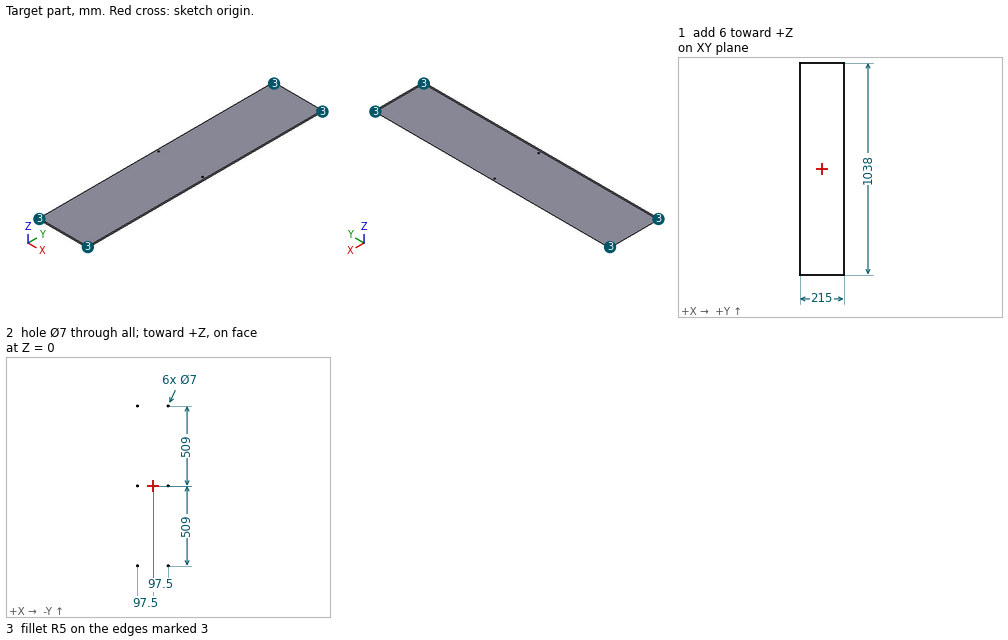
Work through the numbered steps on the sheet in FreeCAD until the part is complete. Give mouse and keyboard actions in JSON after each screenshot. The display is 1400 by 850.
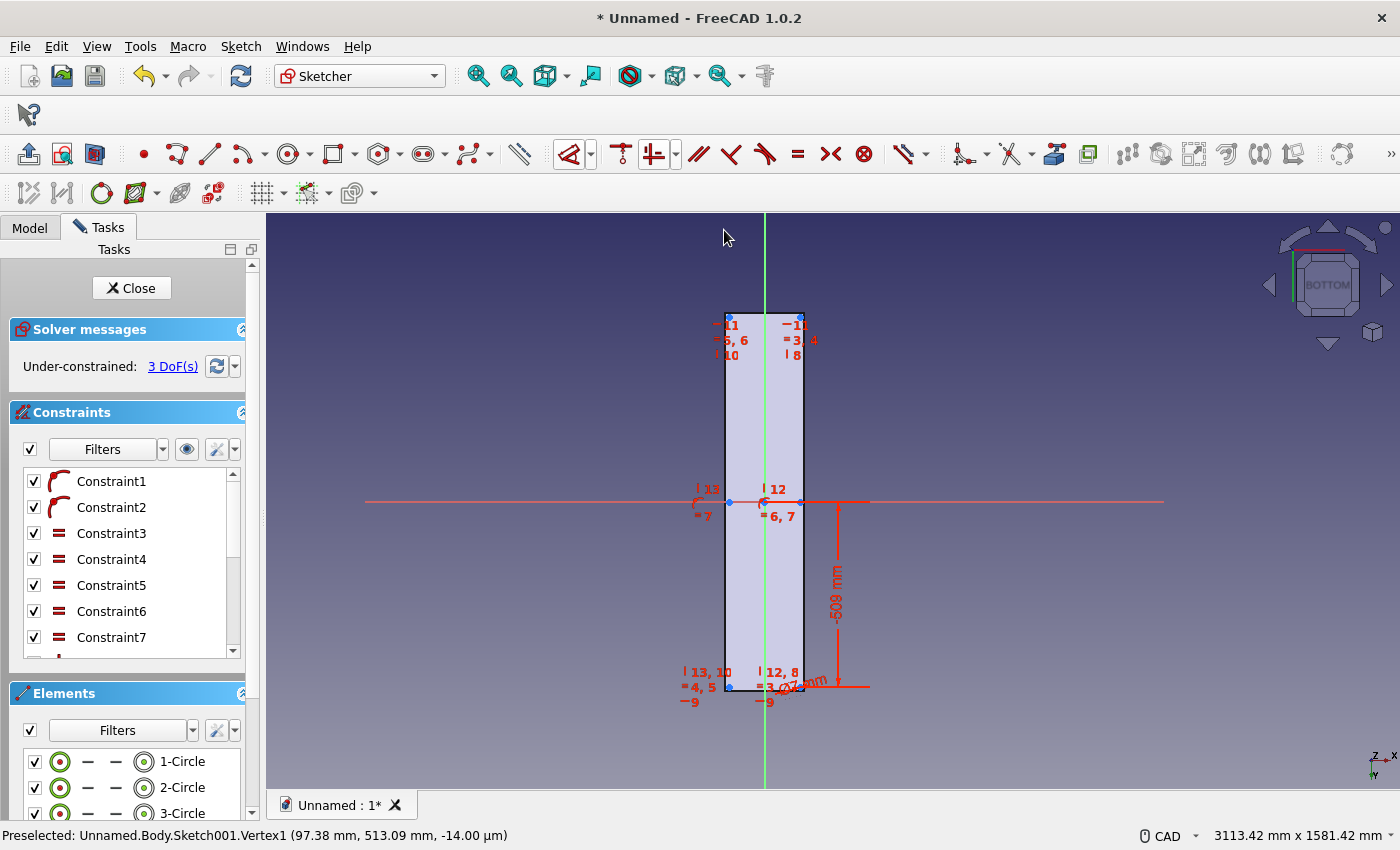
{"action": "left_click", "coordinate": [800, 318]}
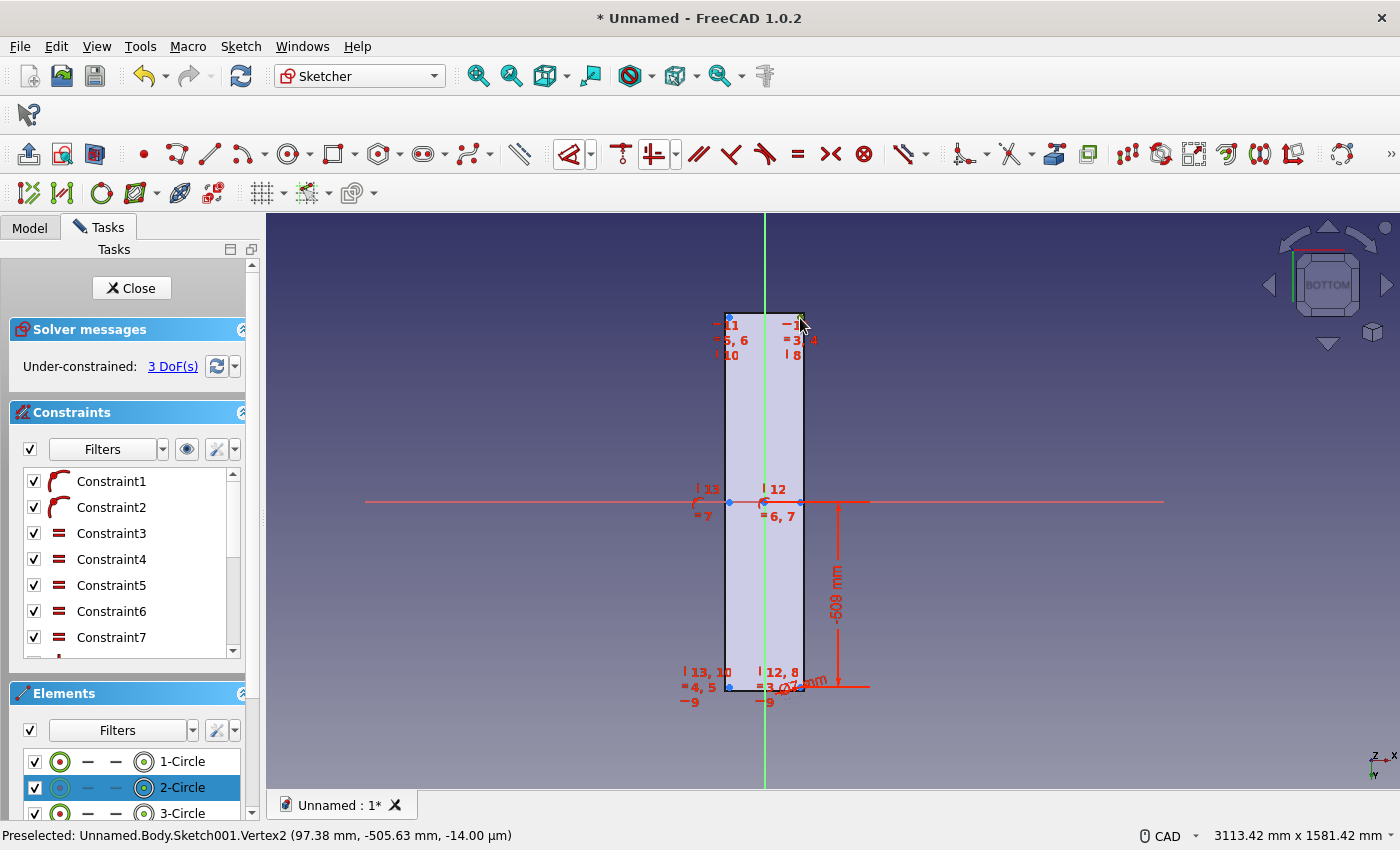
{"action": "key", "text": "i"}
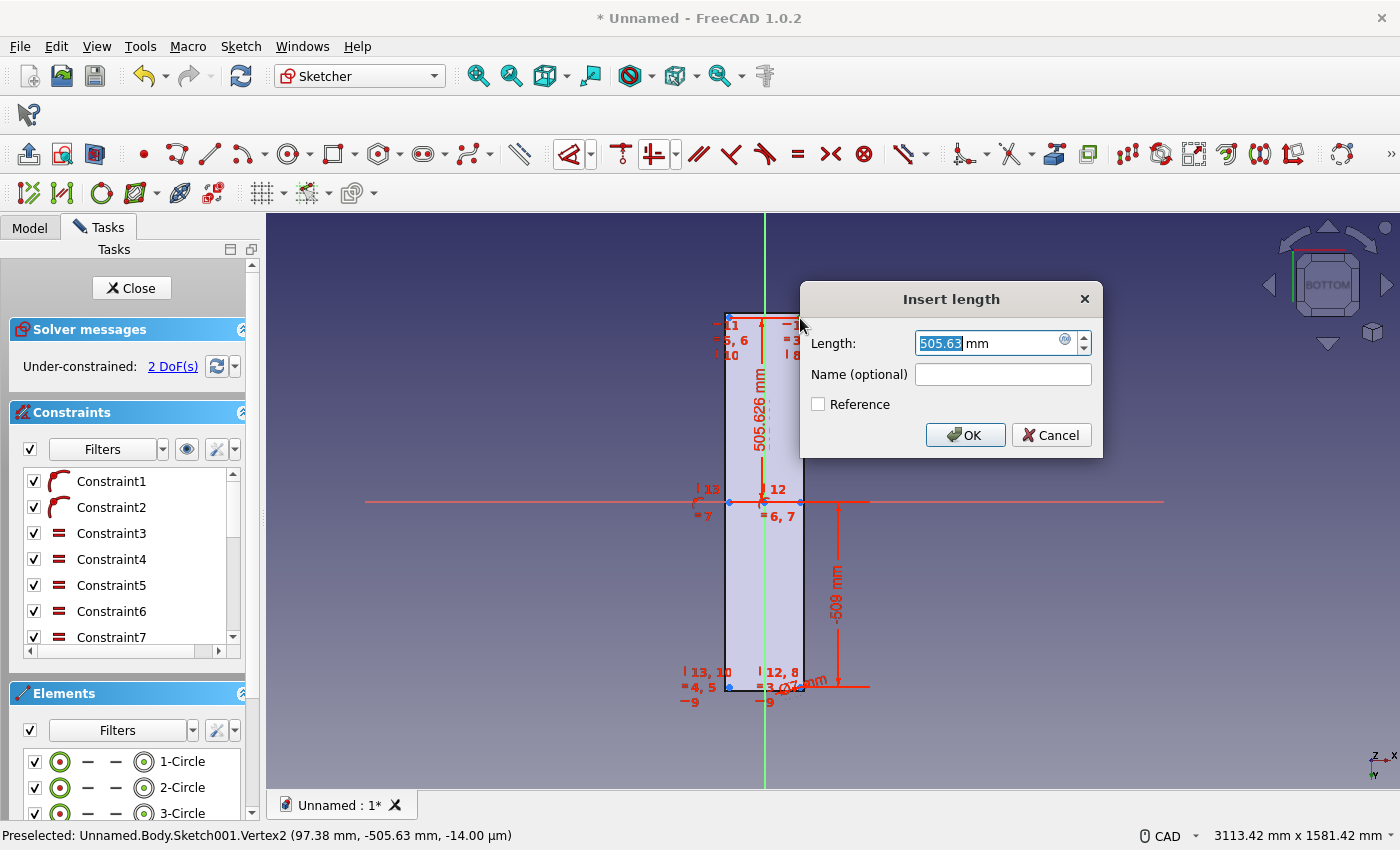
{"action": "type", "text": "509"}
{"action": "key", "text": "Return"}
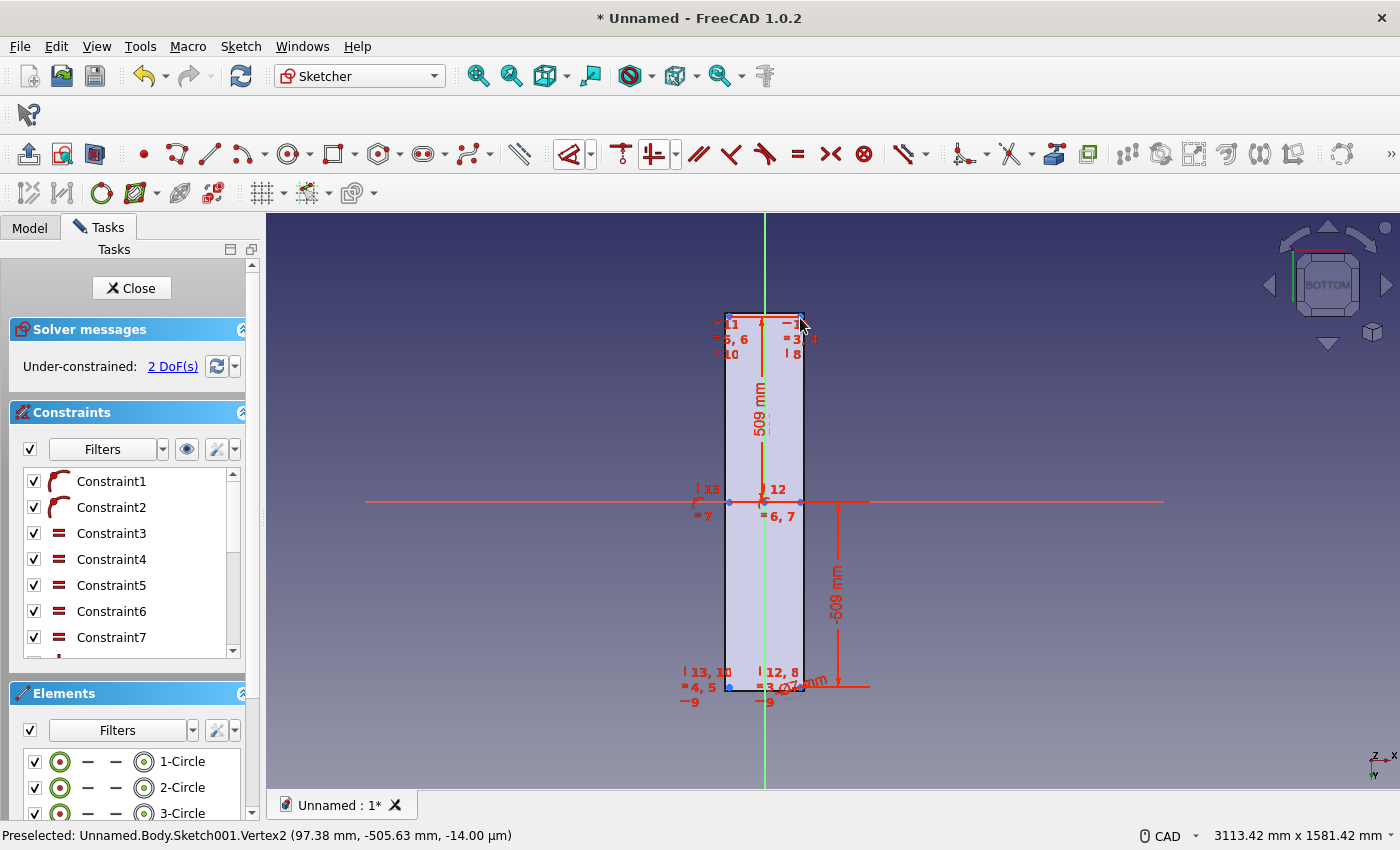
{"action": "left_click", "coordinate": [800, 687]}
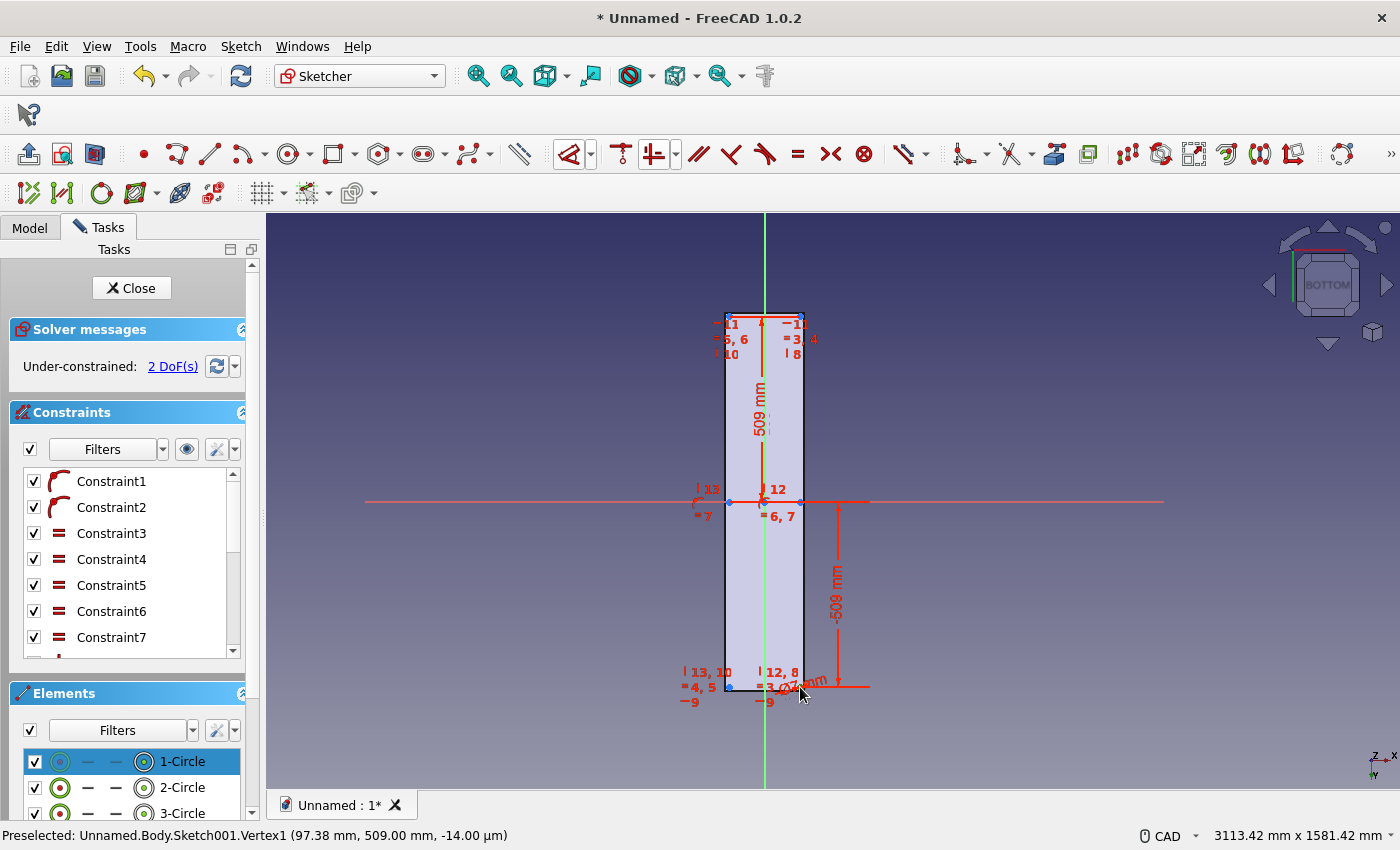
{"action": "key", "text": "l"}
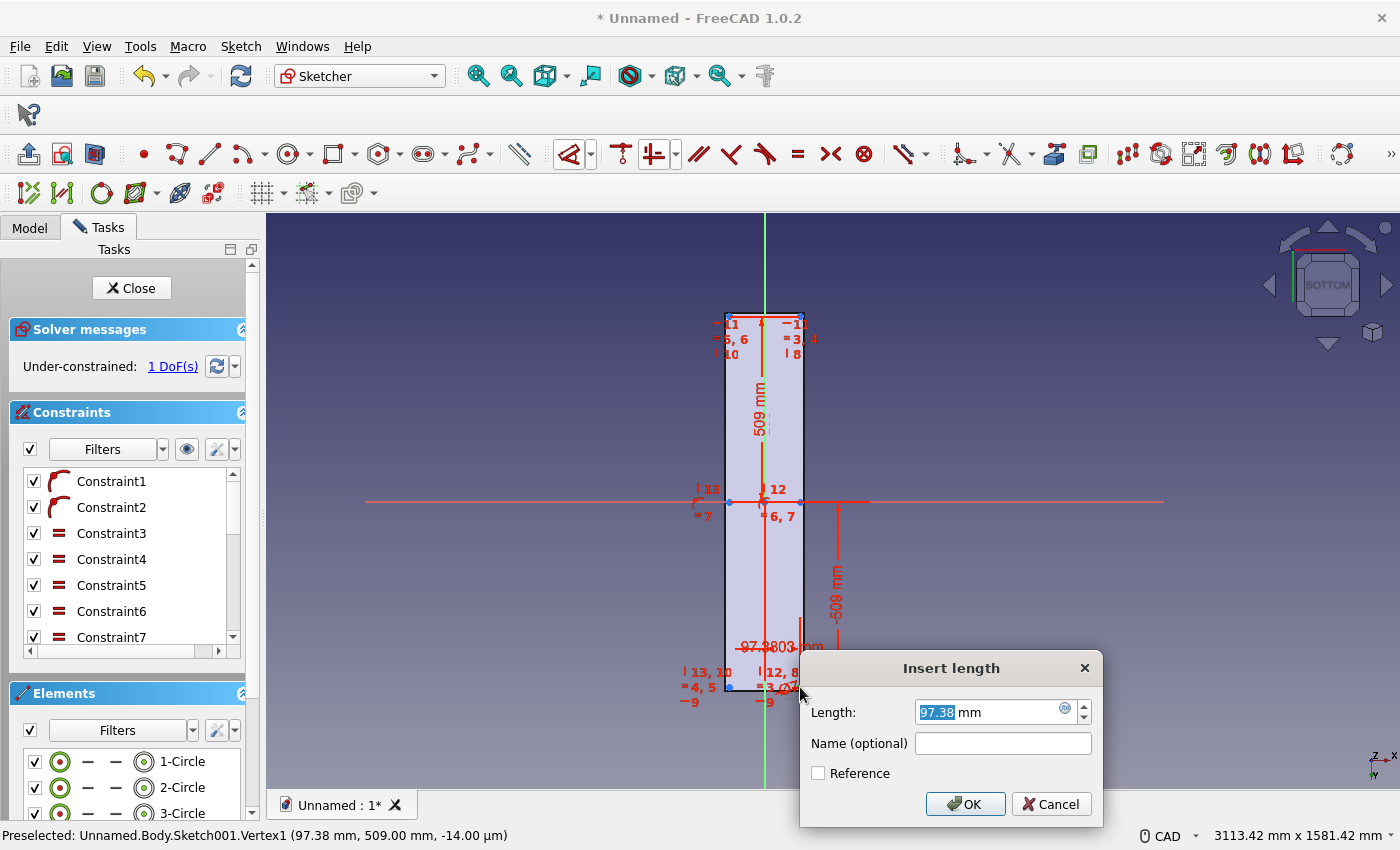
{"action": "type", "text": "97.5"}
{"action": "key", "text": "Return"}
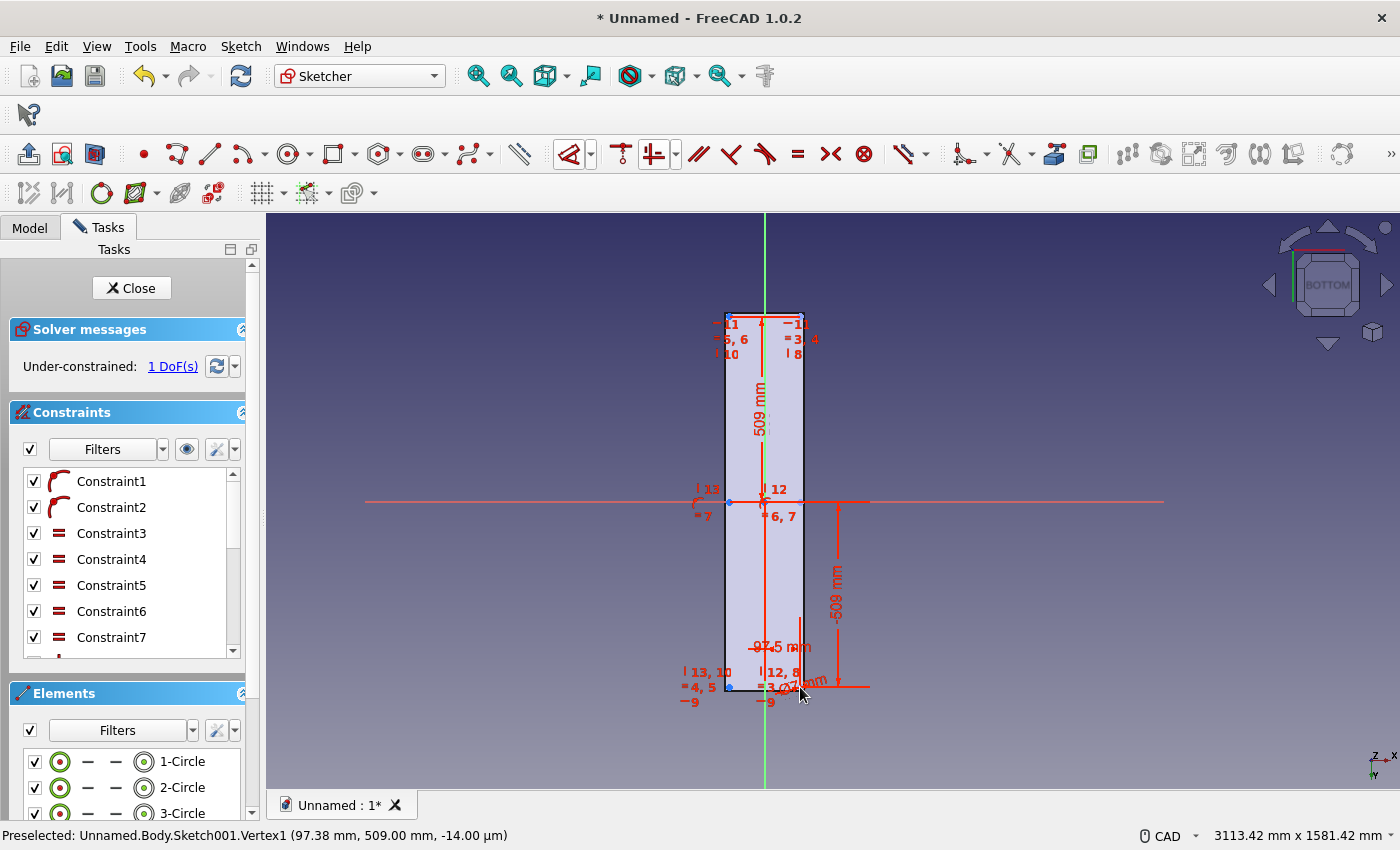
{"action": "left_click", "coordinate": [729, 687]}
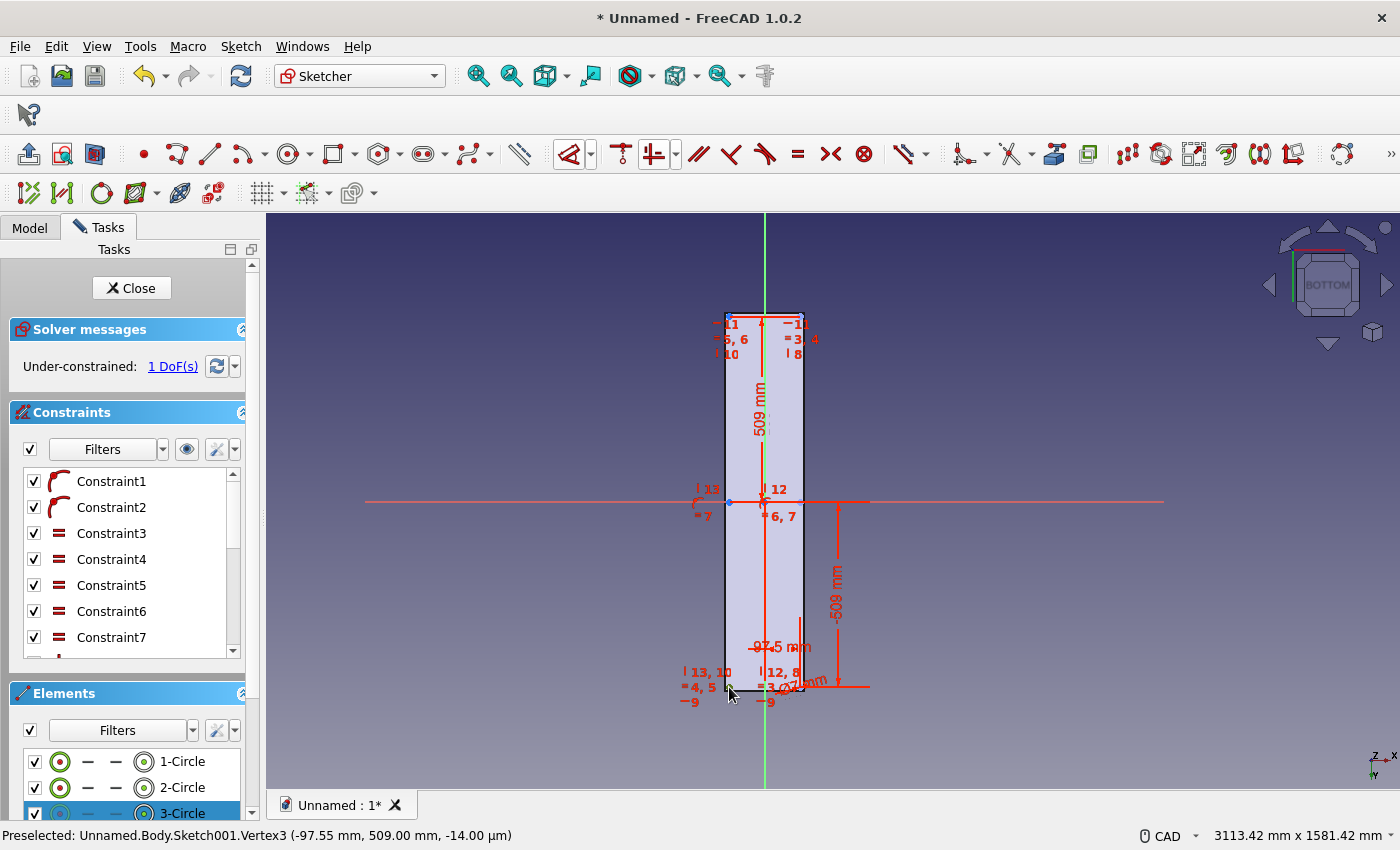
{"action": "key", "text": "l"}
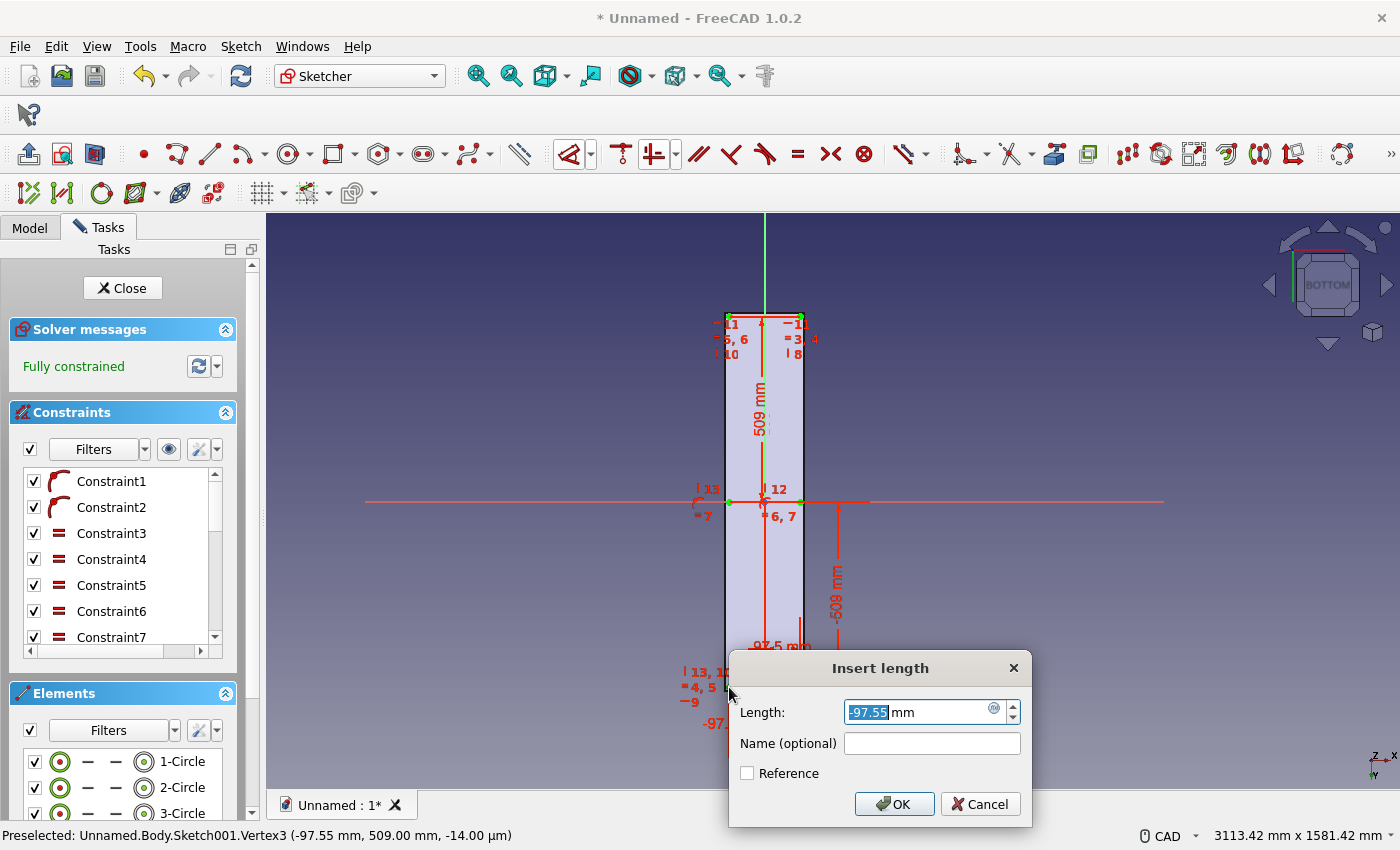
{"action": "type", "text": "-97.5"}
{"action": "key", "text": "Return"}